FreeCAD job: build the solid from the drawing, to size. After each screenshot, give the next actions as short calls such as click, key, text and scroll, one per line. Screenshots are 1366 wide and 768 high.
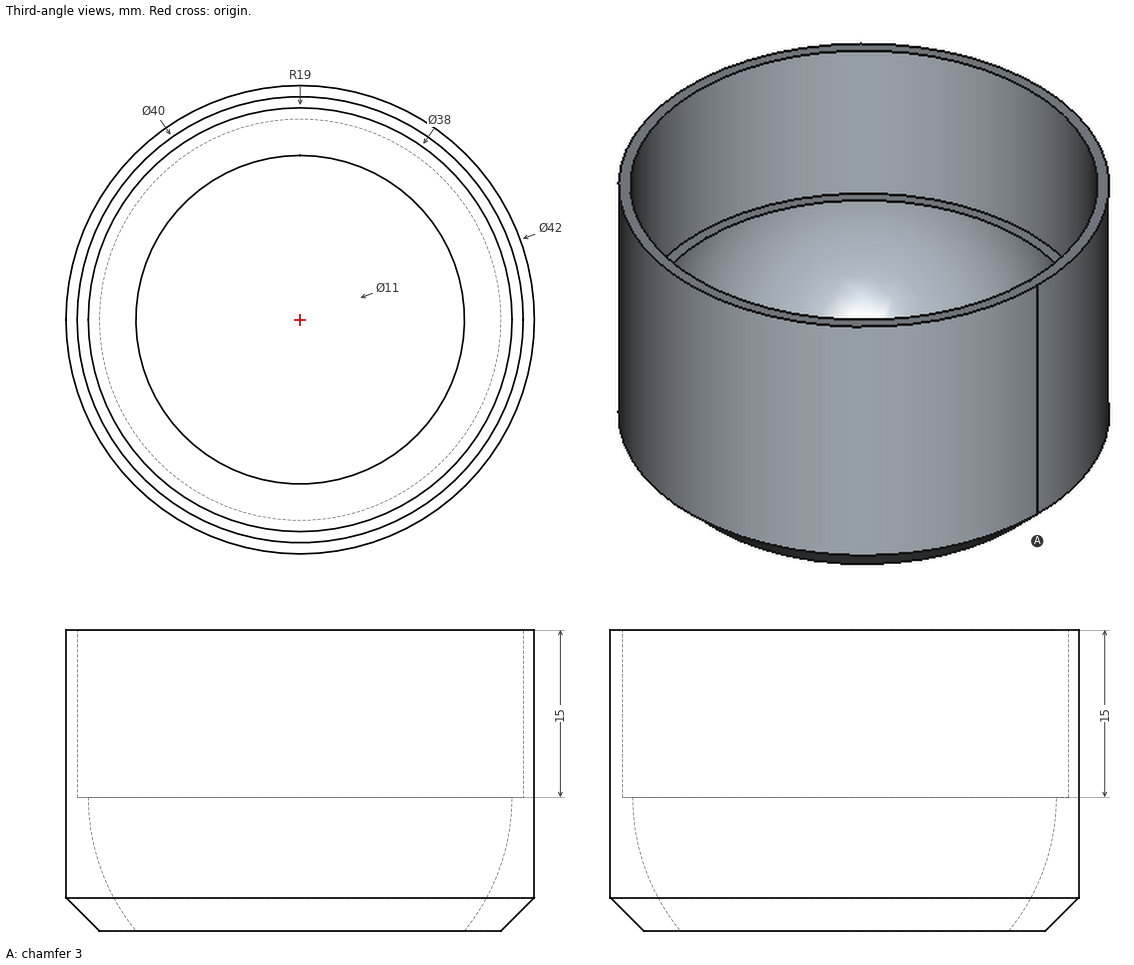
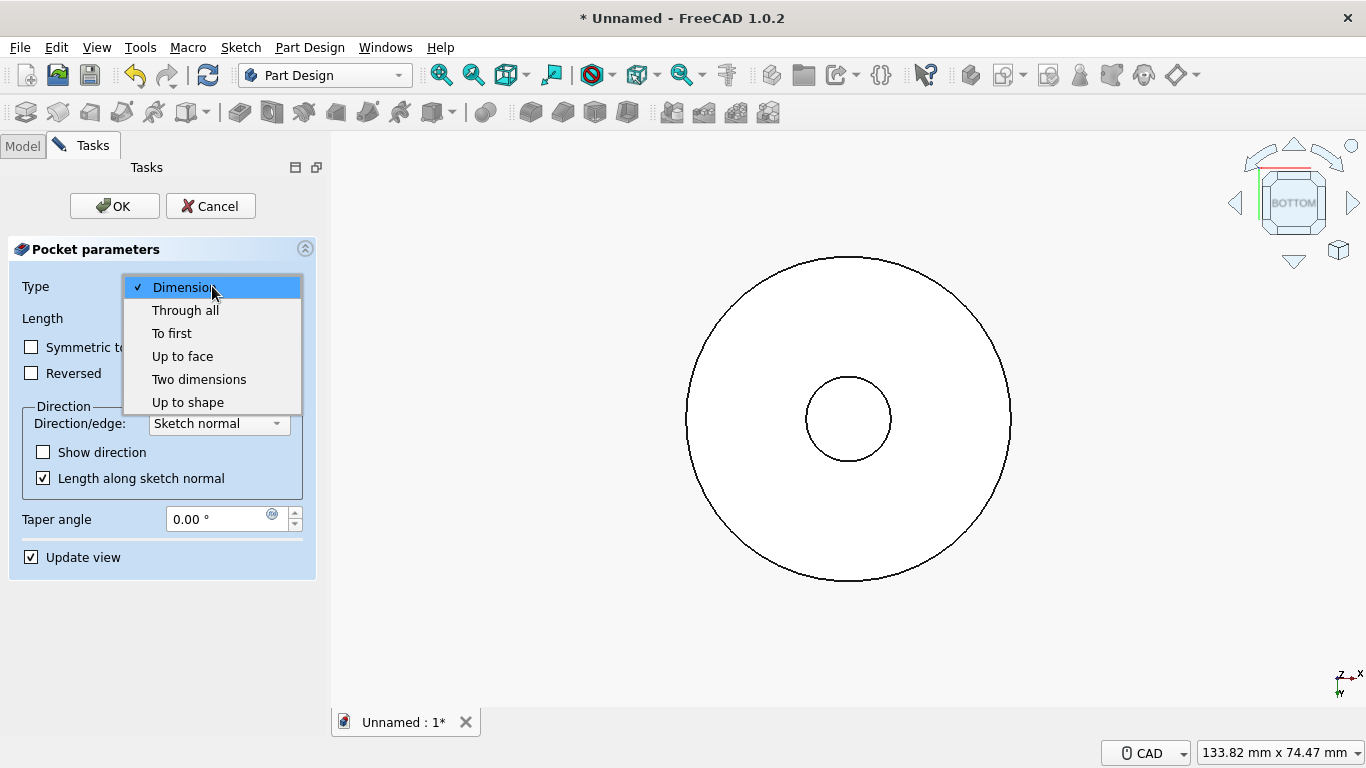
click(212, 310)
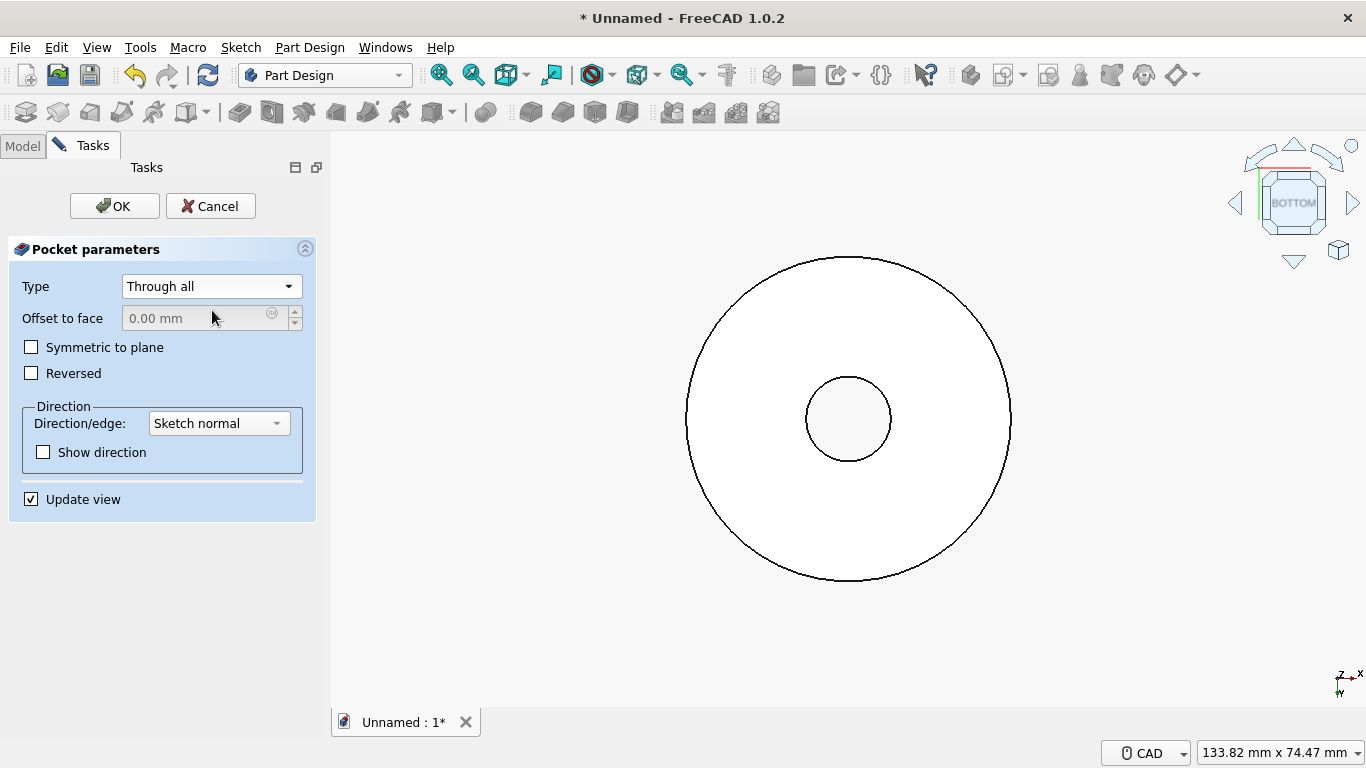
click(115, 206)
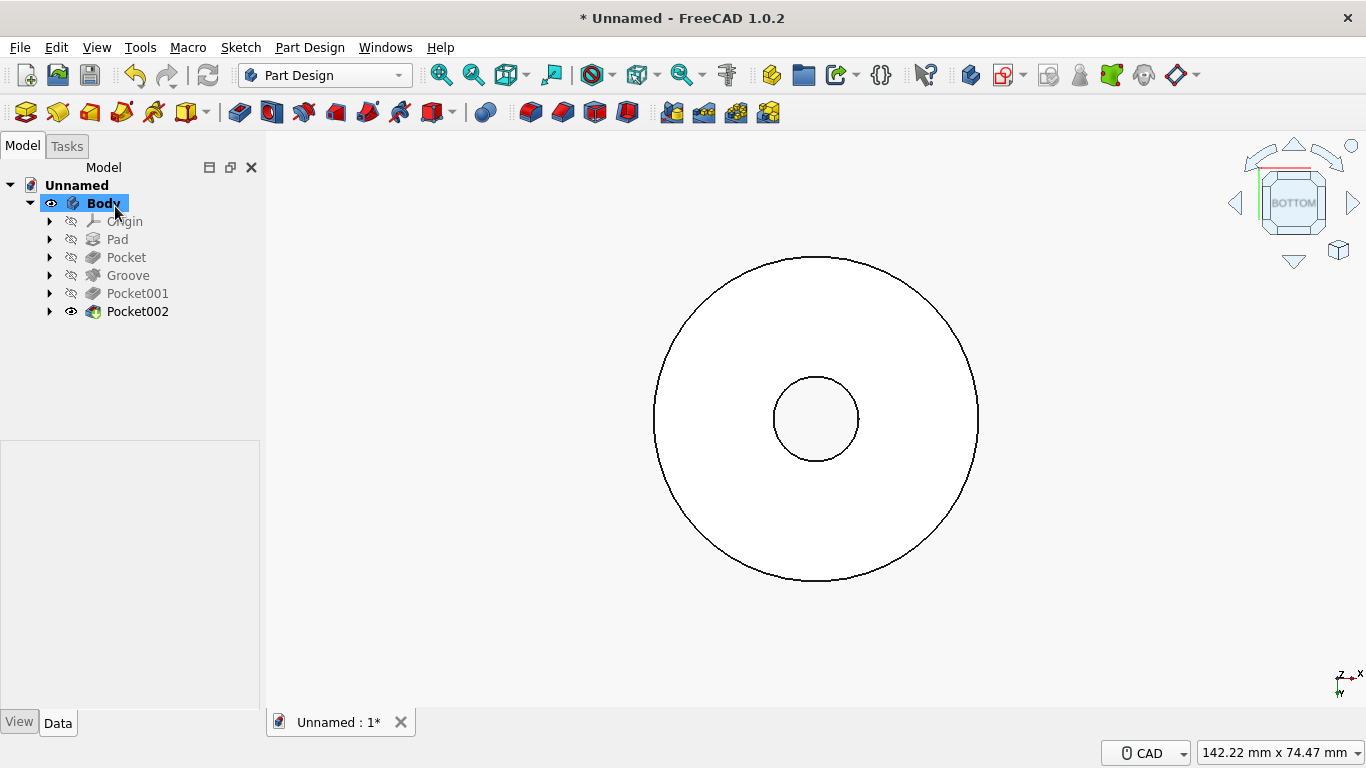
click(1004, 76)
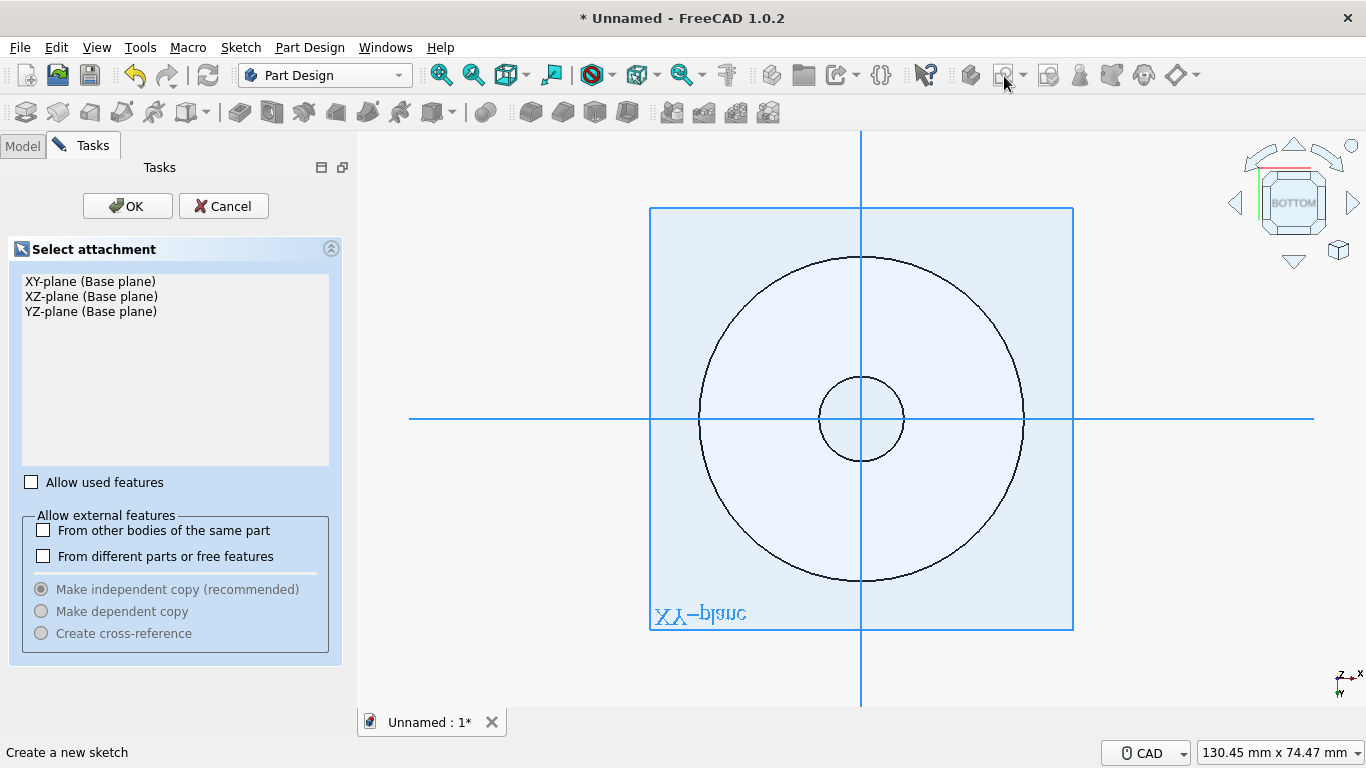
click(82, 282)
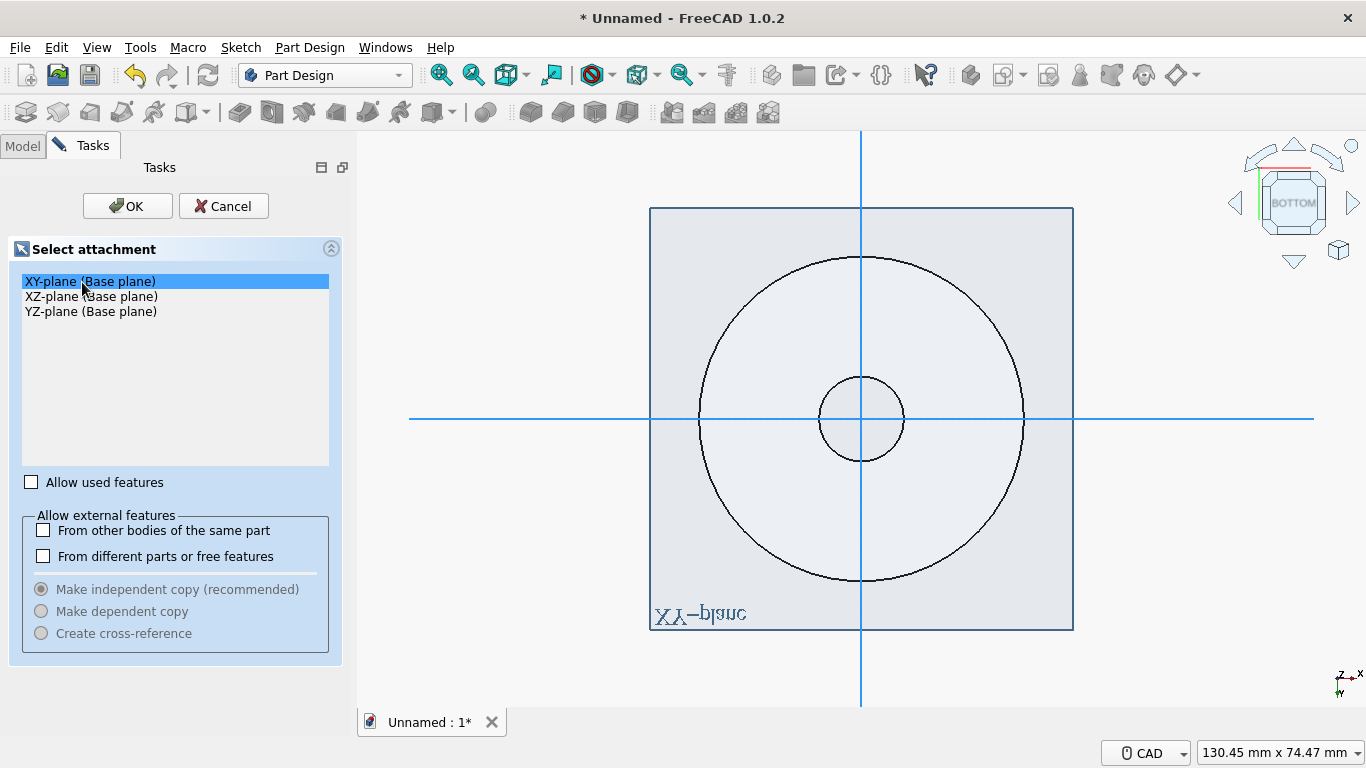
click(128, 206)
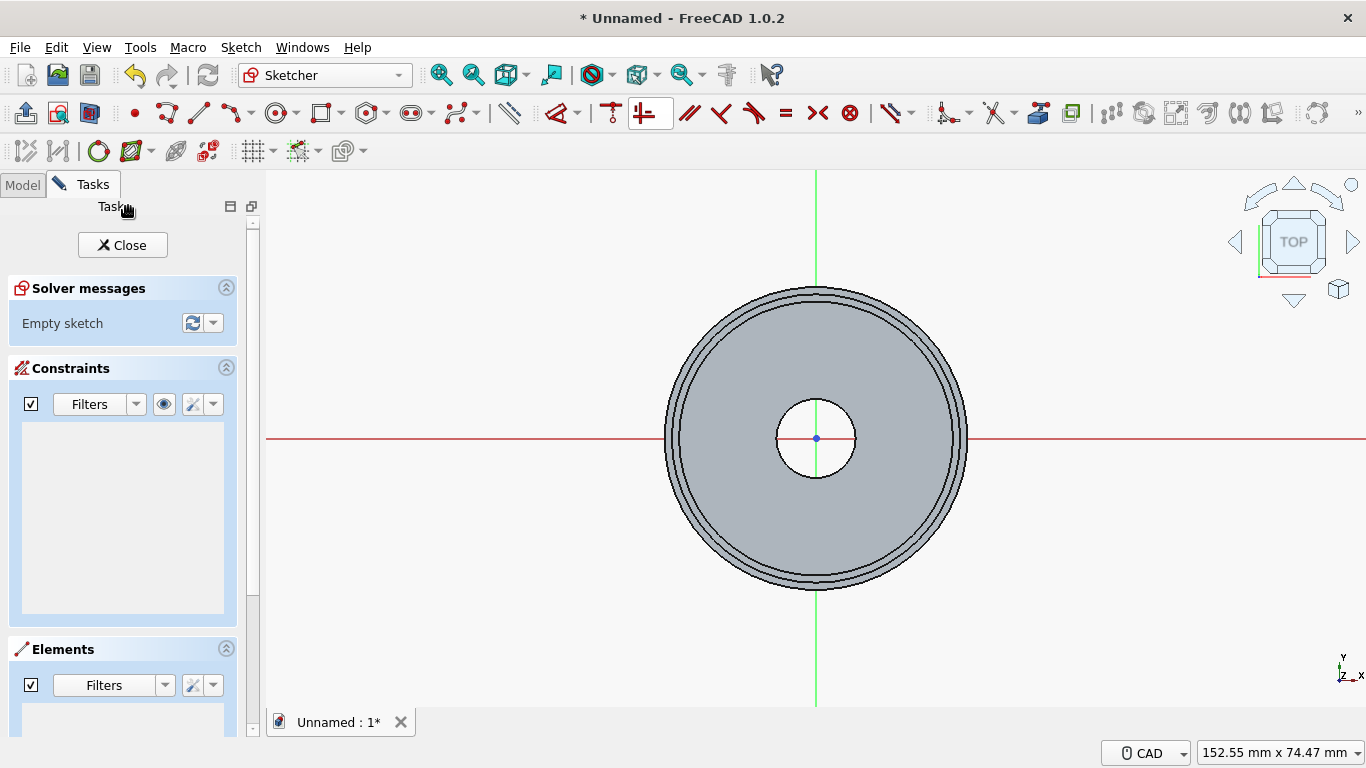
click(90, 114)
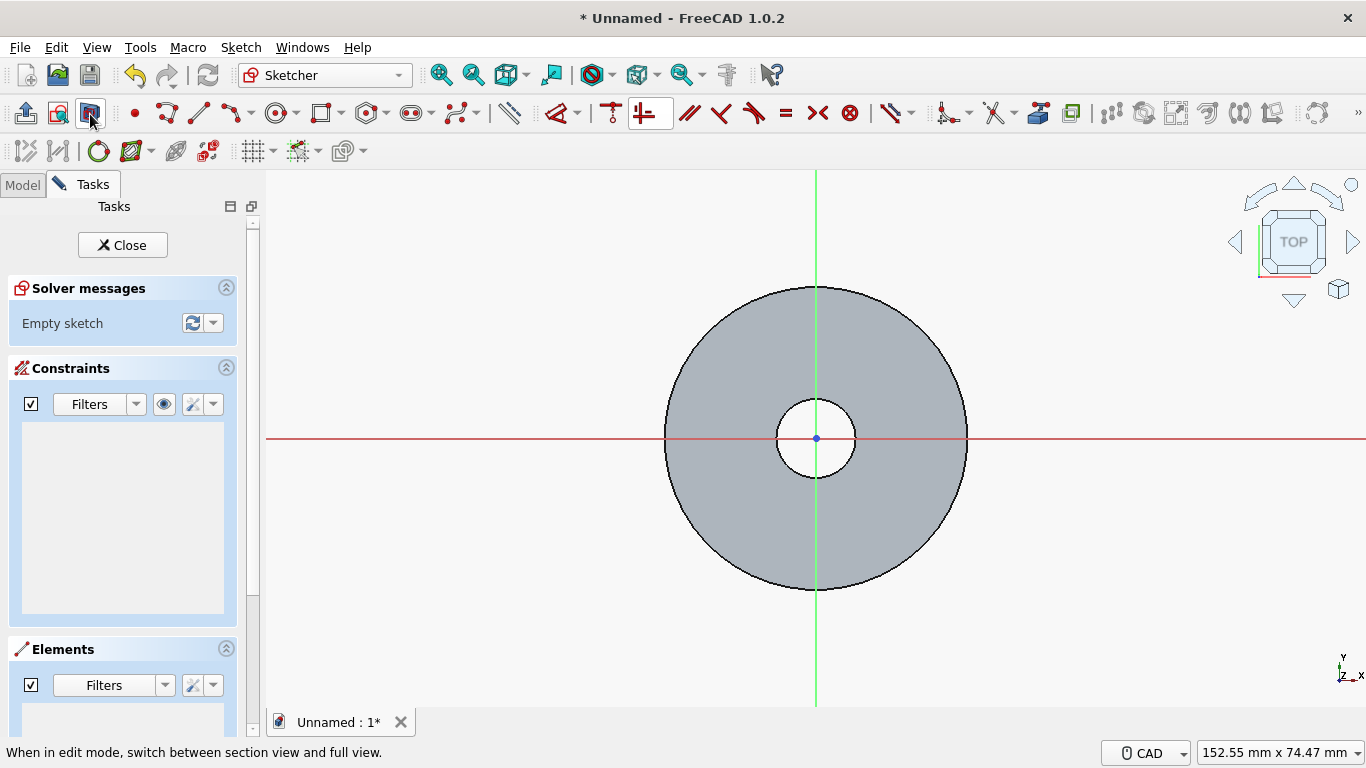
click(276, 114)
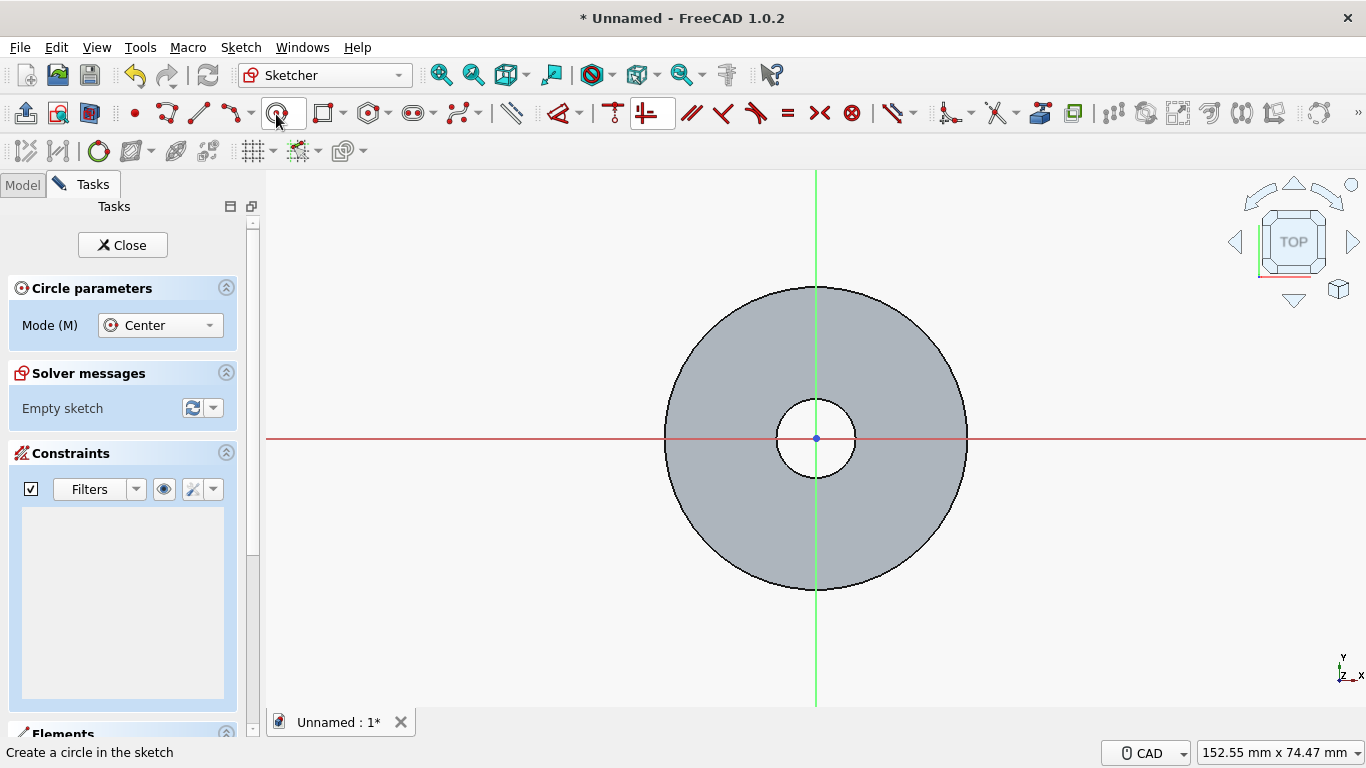
click(816, 438)
move(923, 331)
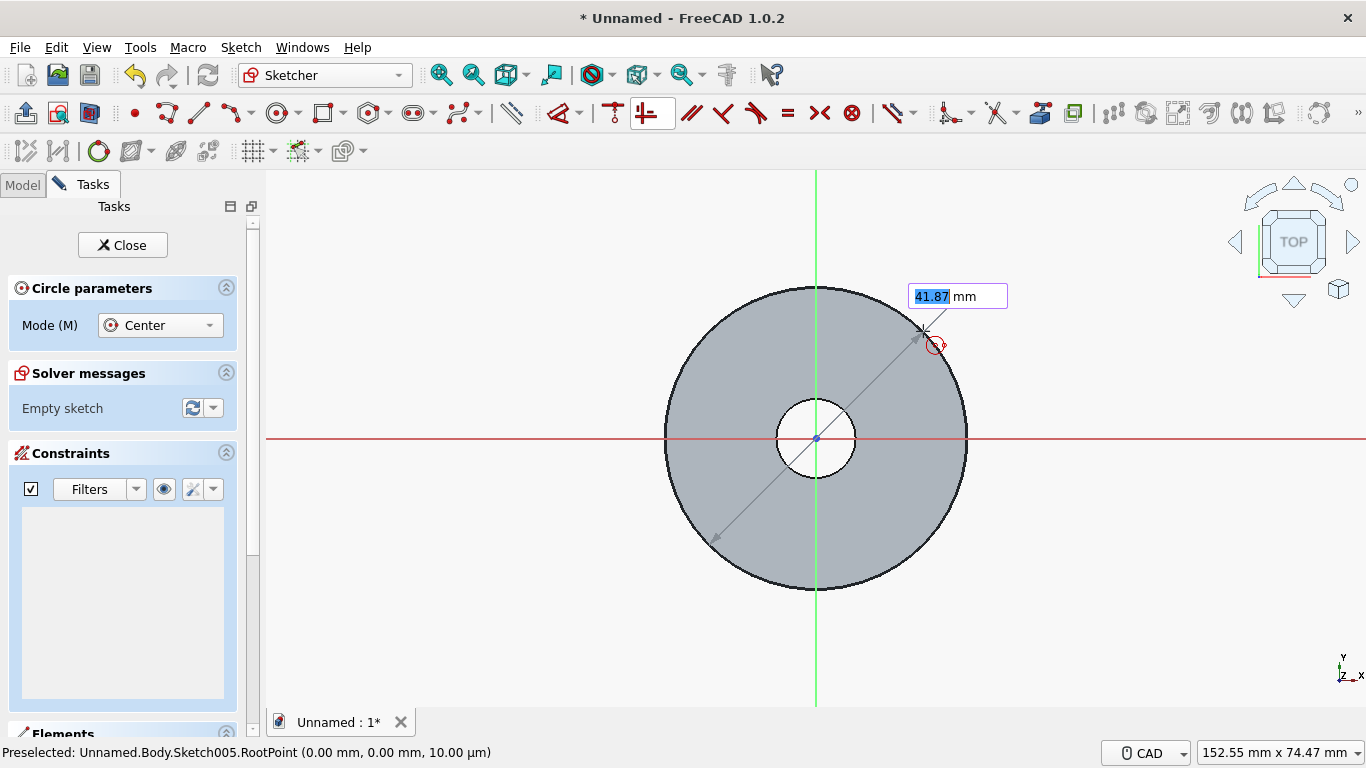
text(42)
key(Return)
key(Escape)